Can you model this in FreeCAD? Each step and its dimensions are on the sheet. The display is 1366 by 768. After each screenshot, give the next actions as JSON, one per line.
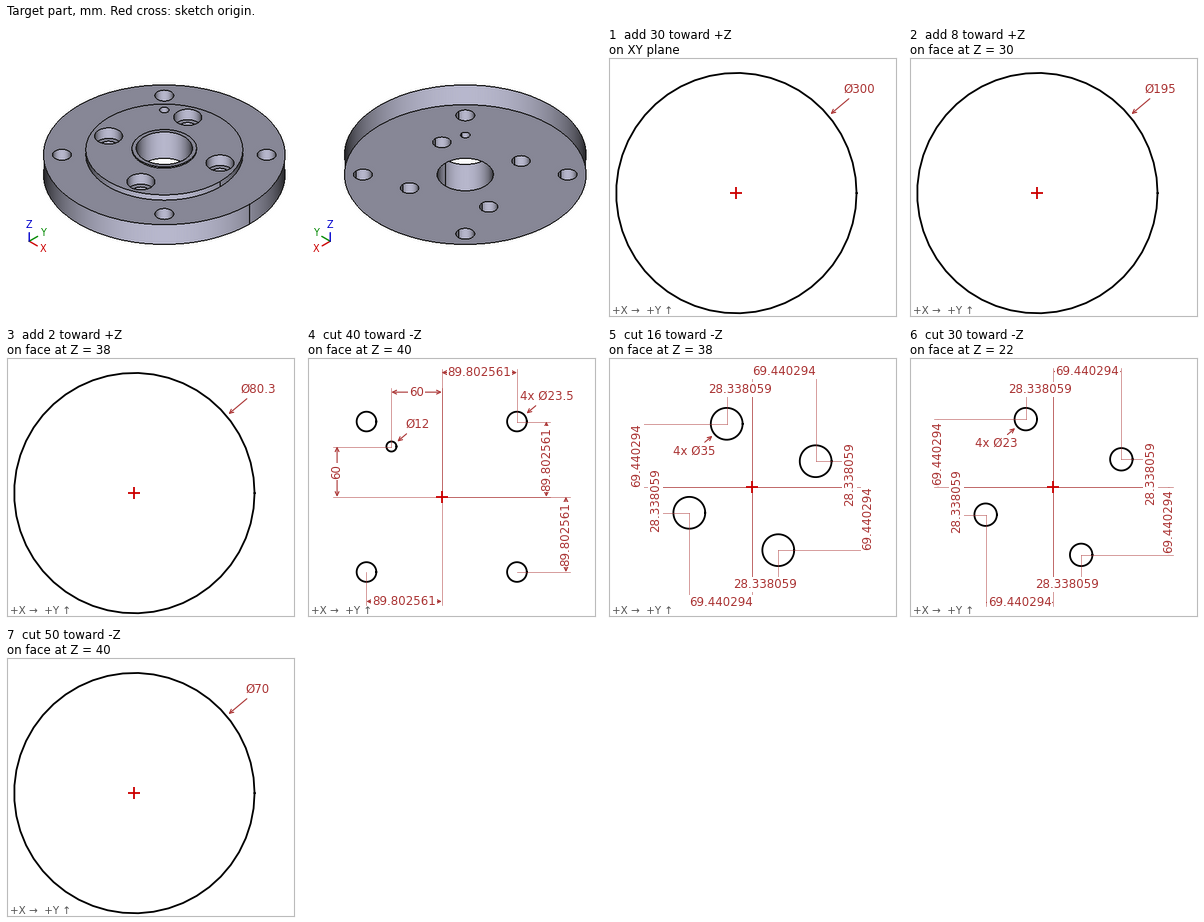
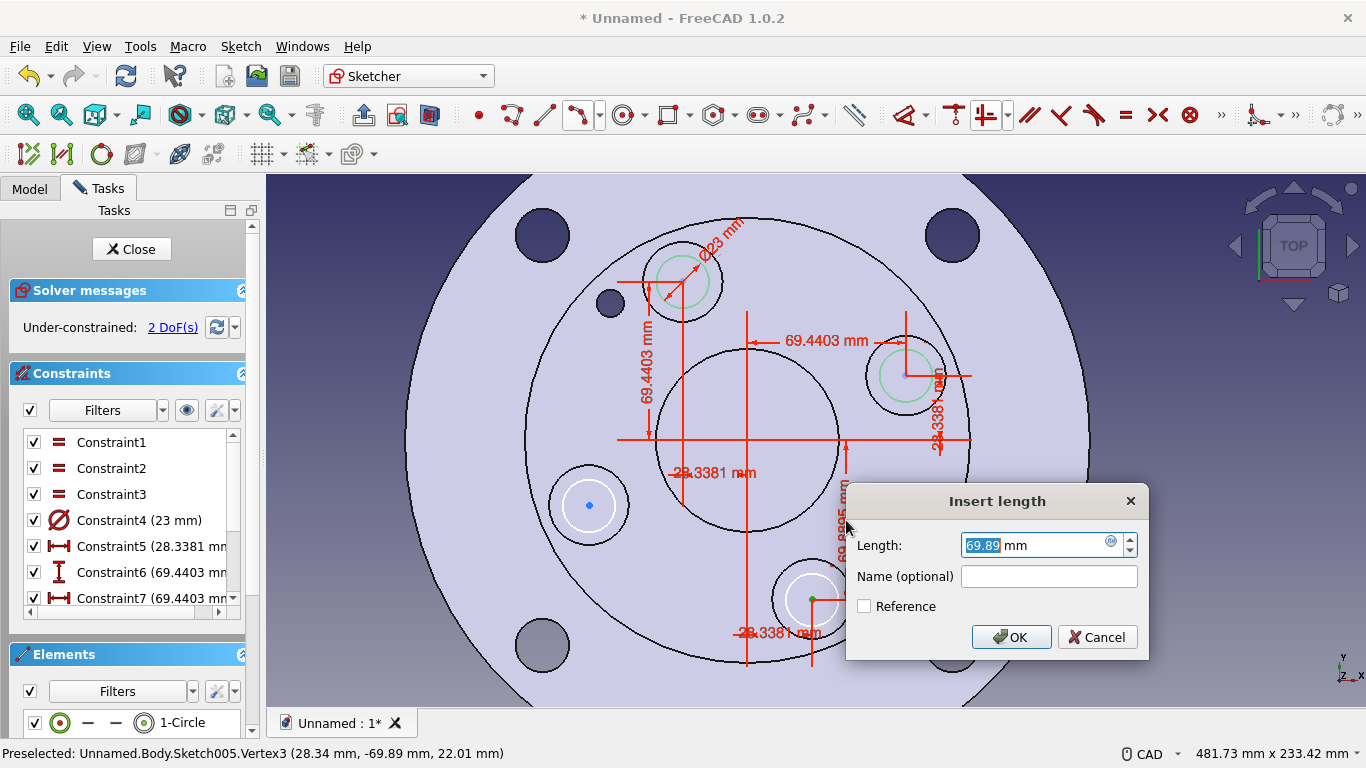
{"action": "type", "text": "69.440294"}
{"action": "key", "text": "Return"}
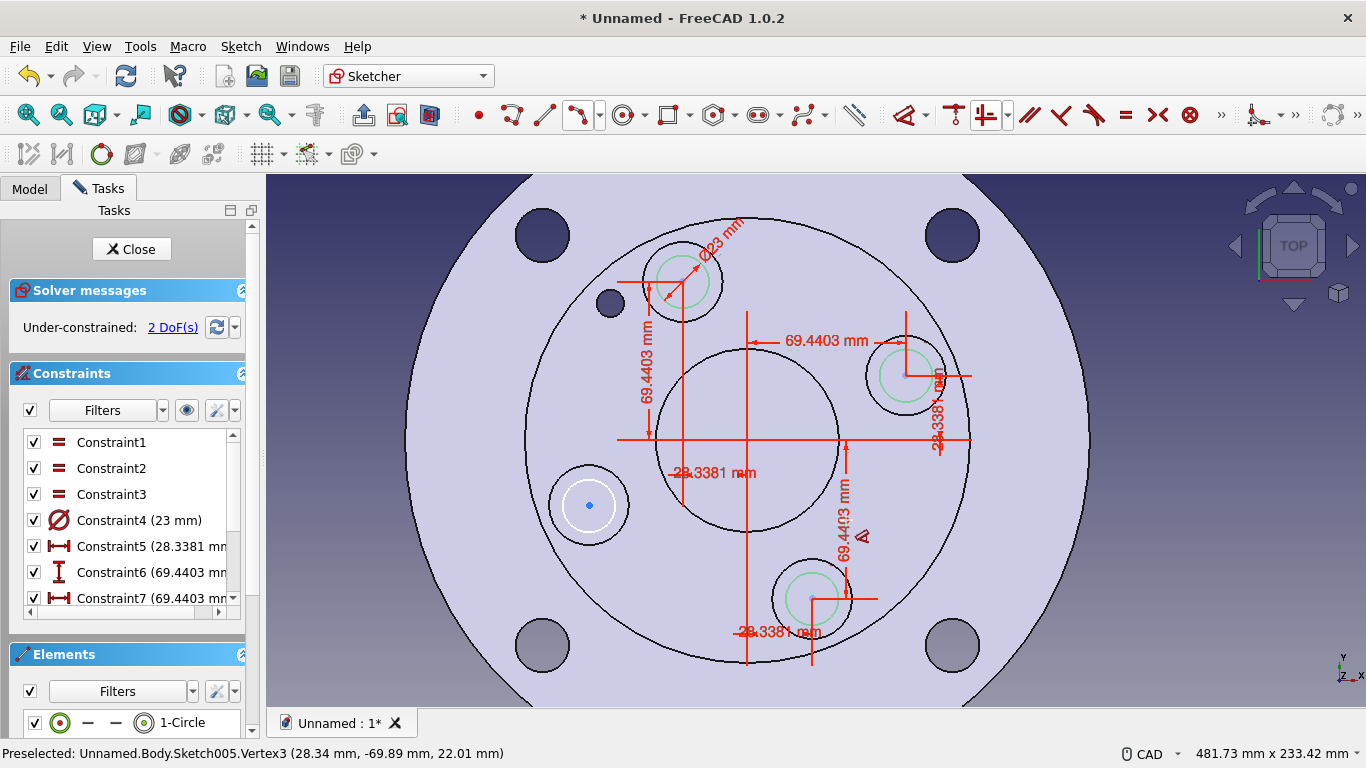
{"action": "left_click", "coordinate": [589, 506]}
{"action": "left_click", "coordinate": [668, 540]}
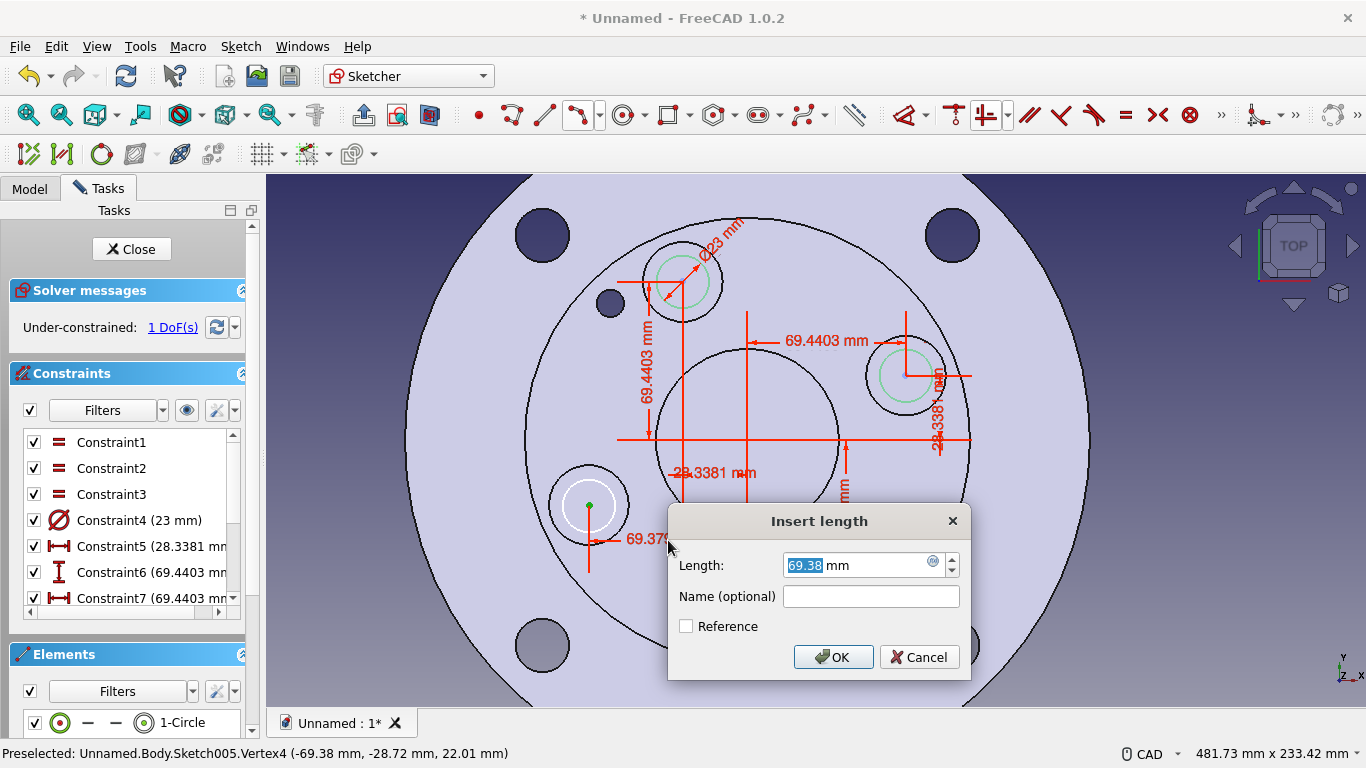
{"action": "type", "text": "69.440294"}
{"action": "key", "text": "Return"}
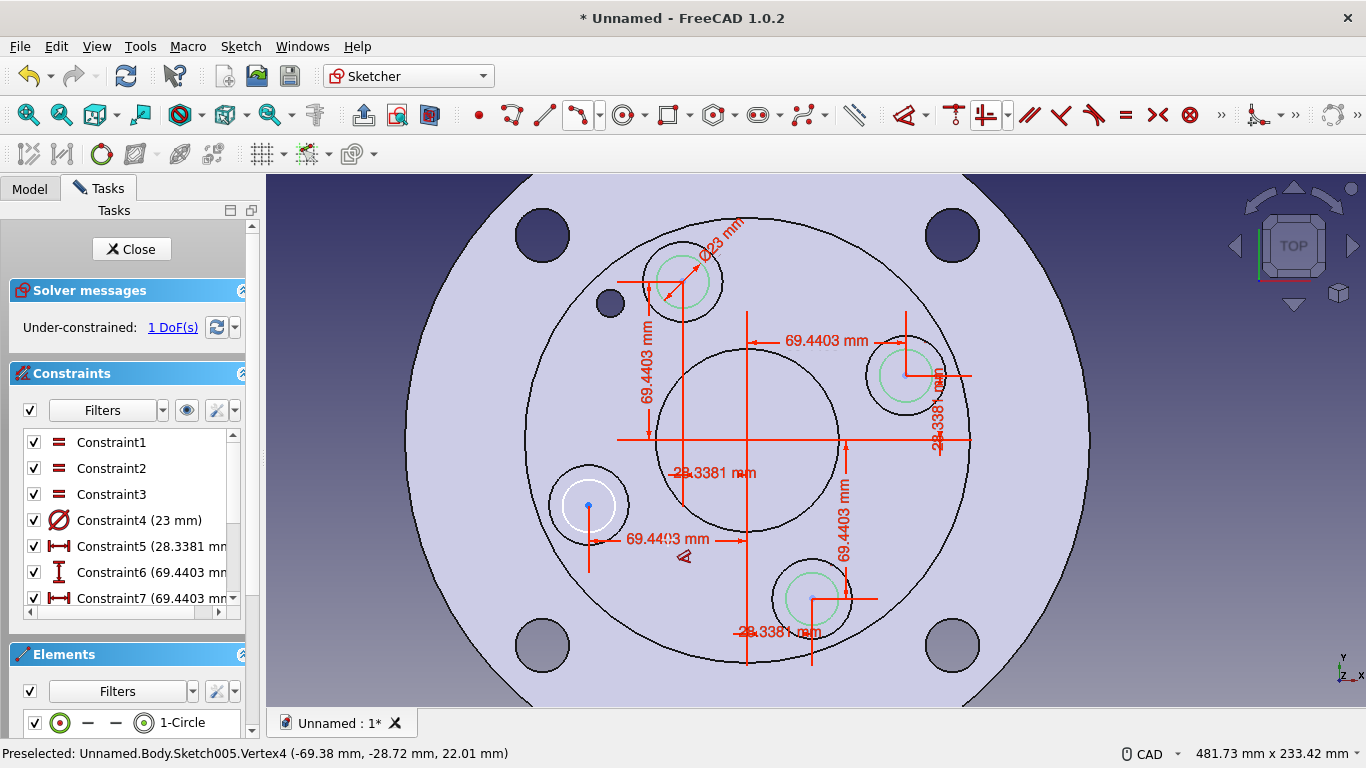
{"action": "left_click", "coordinate": [589, 506]}
{"action": "left_click", "coordinate": [555, 473]}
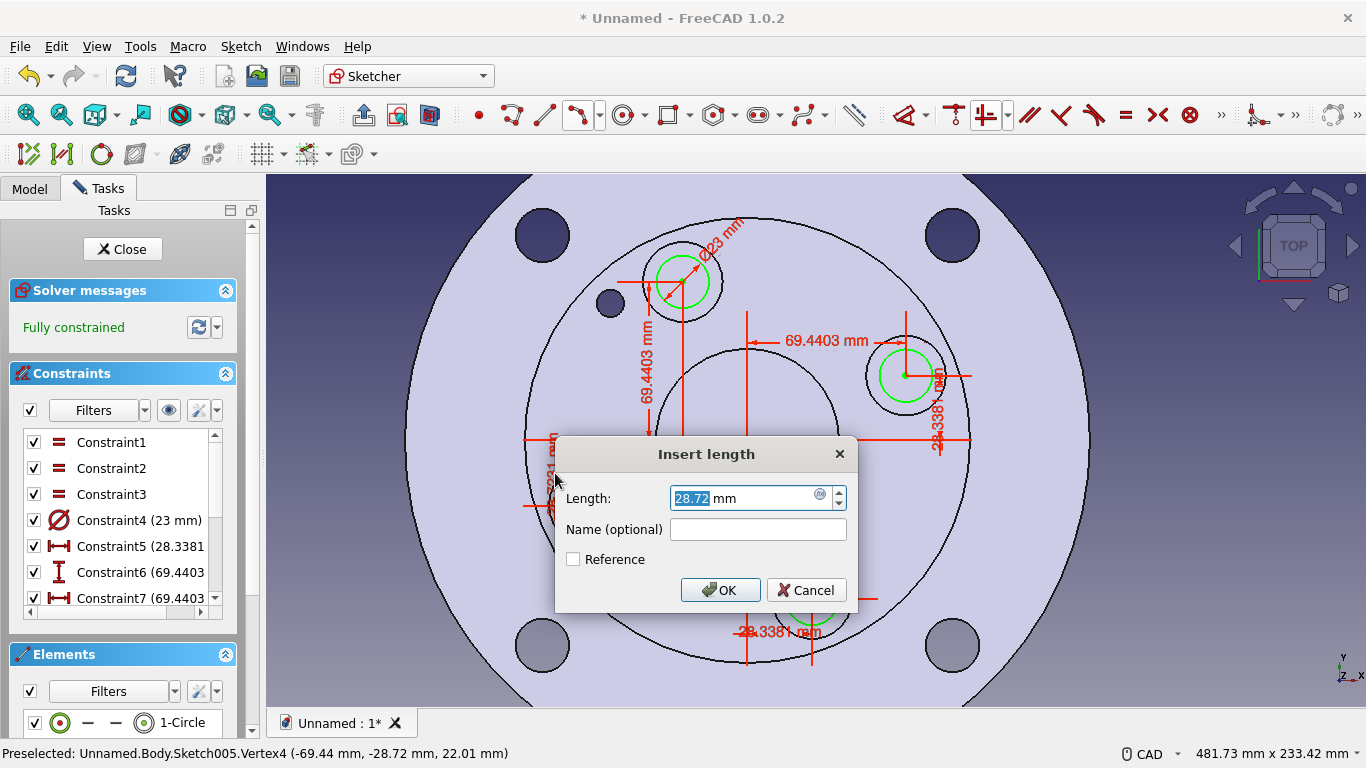
{"action": "type", "text": "28.338059"}
{"action": "key", "text": "Return"}
{"action": "key", "text": "Escape"}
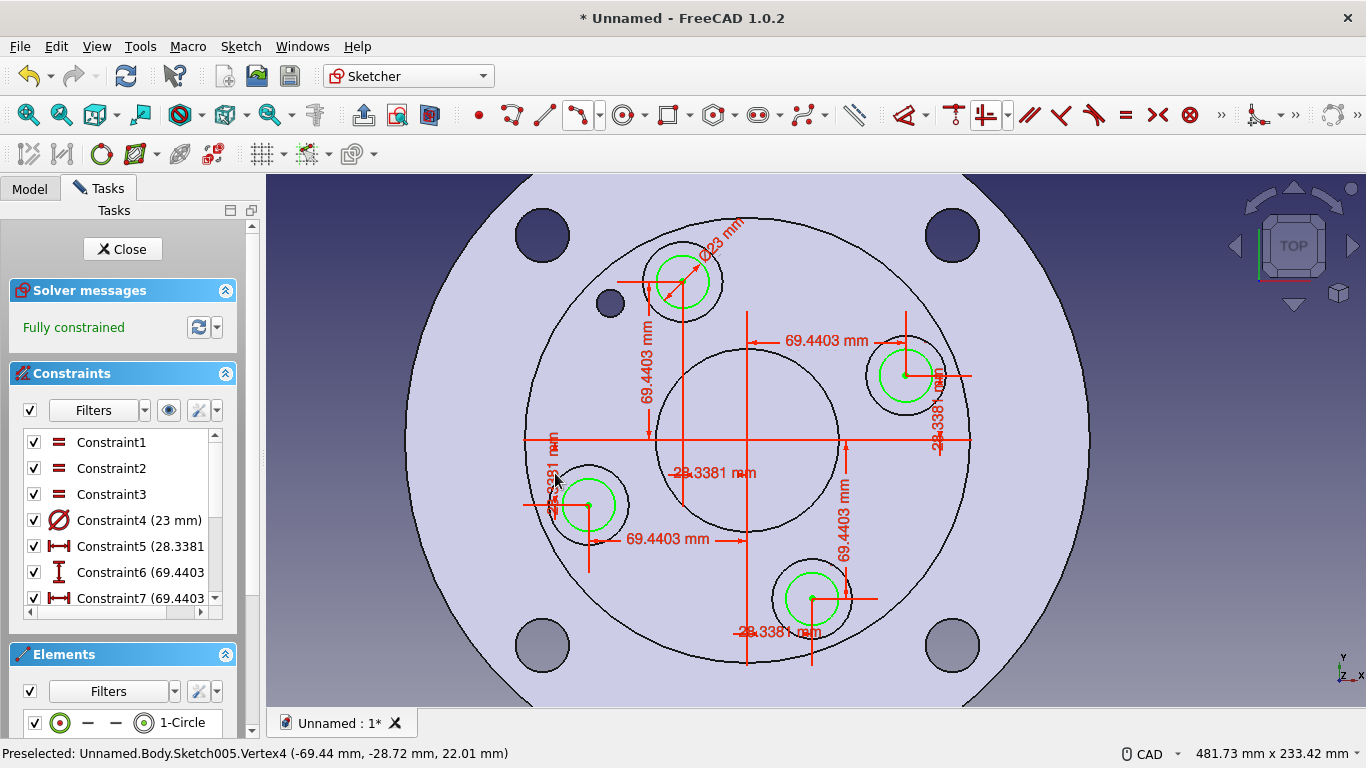
{"action": "left_click", "coordinate": [123, 249]}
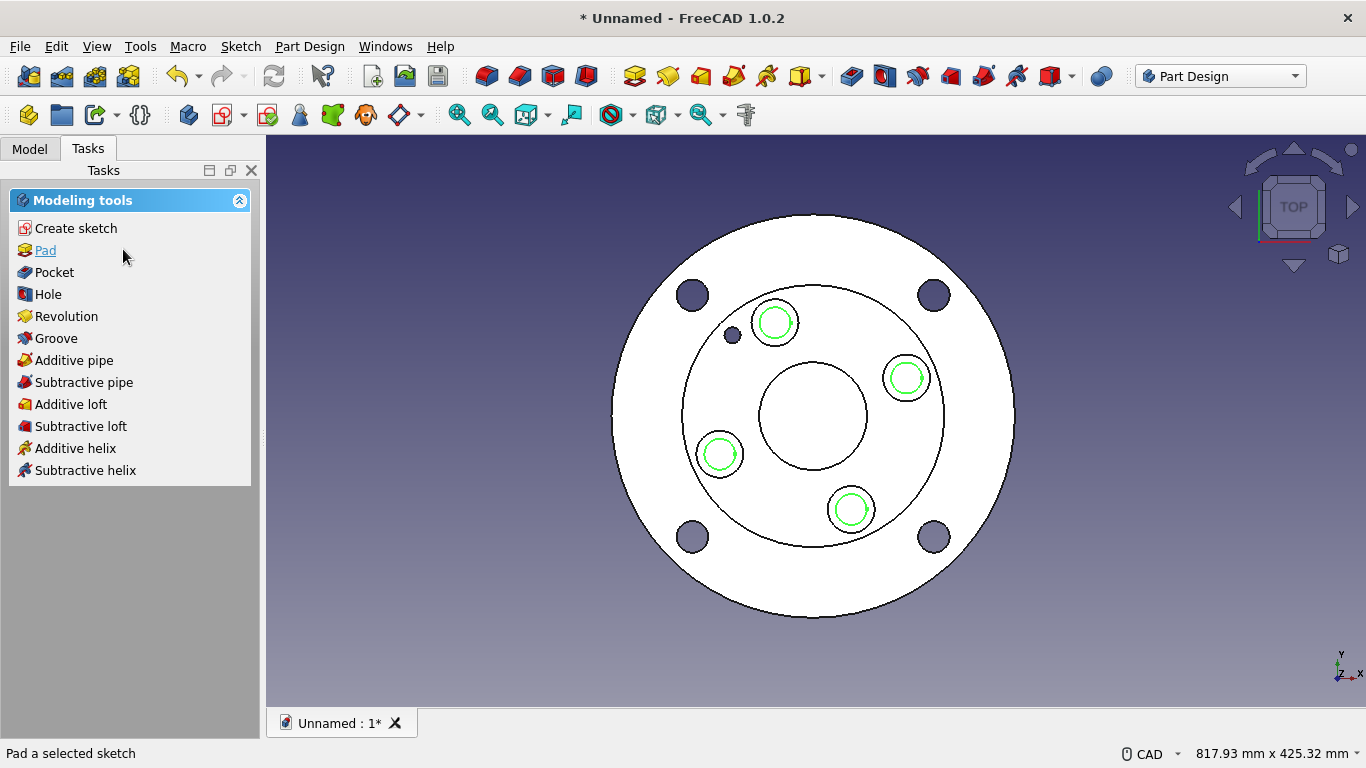
{"action": "left_click", "coordinate": [852, 76]}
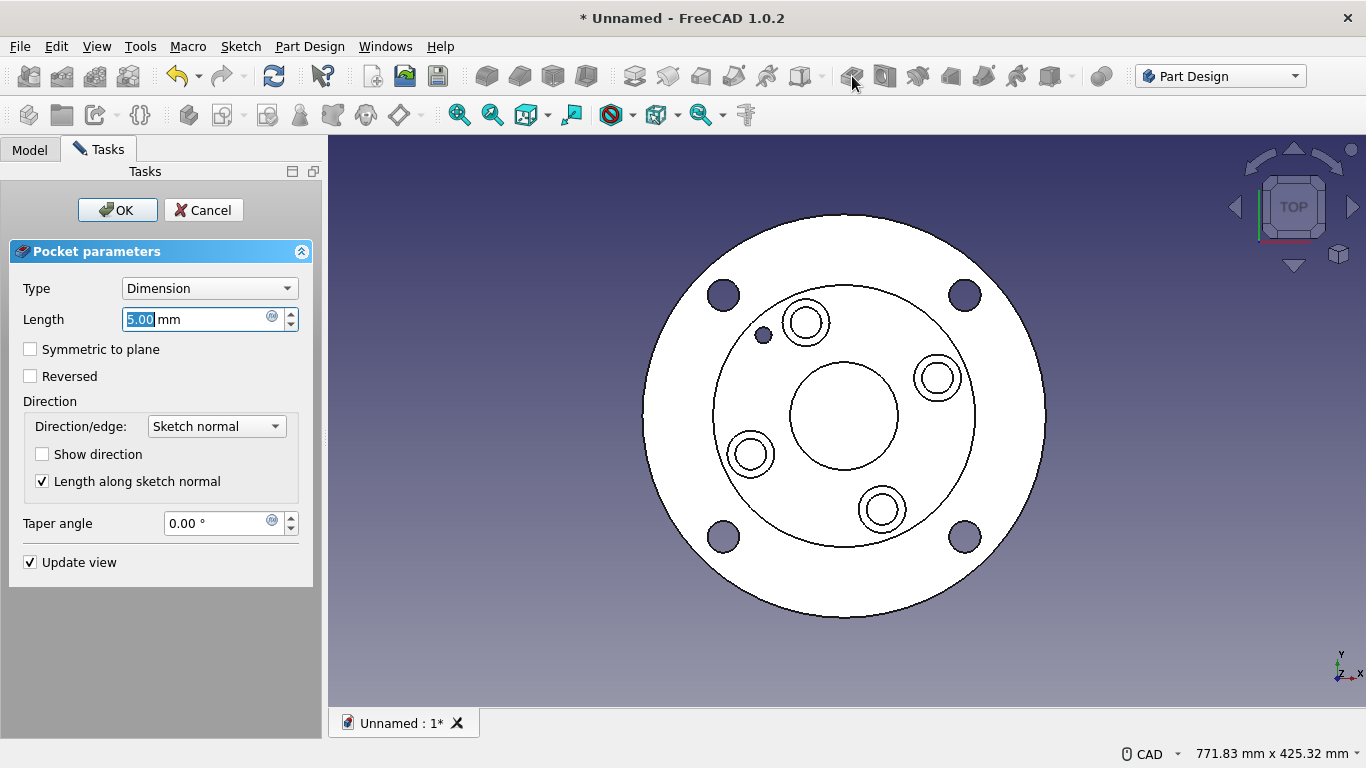
{"action": "type", "text": "30"}
{"action": "key", "text": "Tab"}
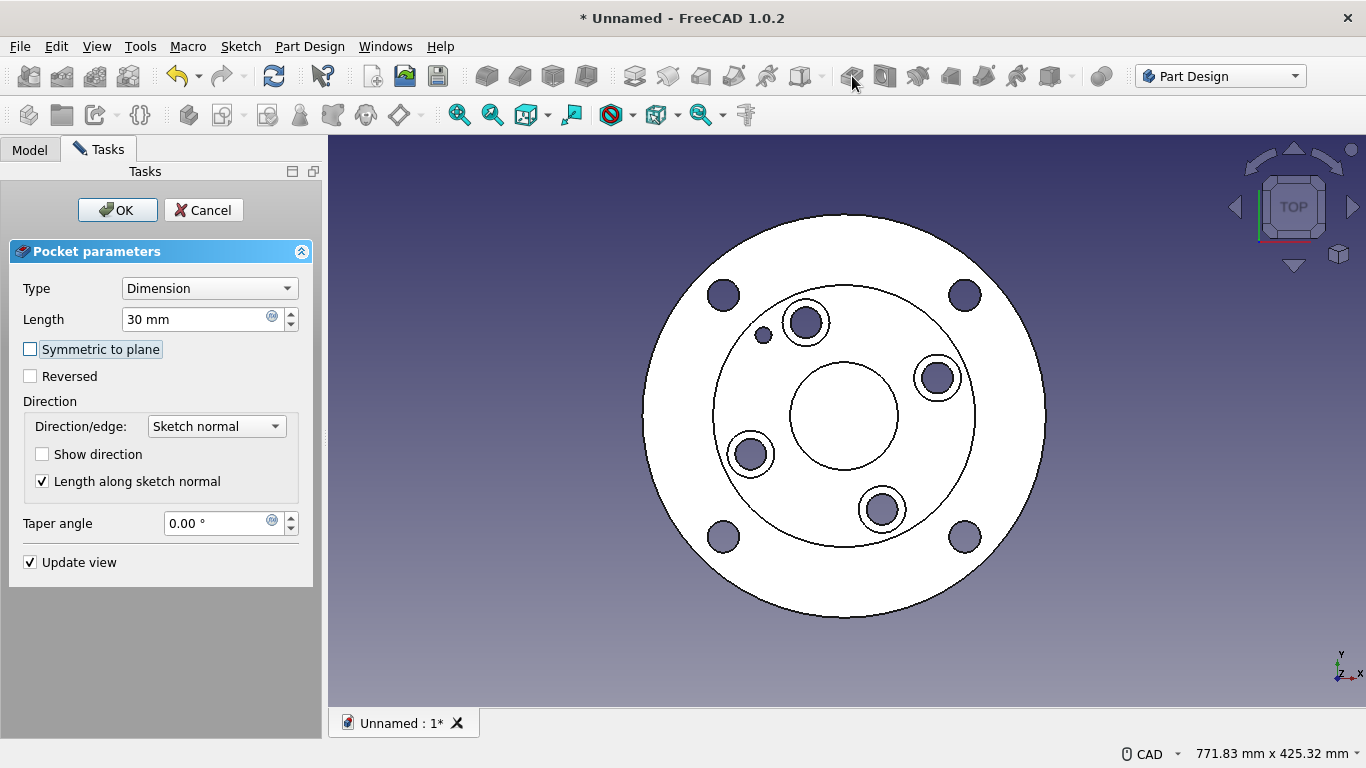
{"action": "left_click", "coordinate": [118, 210]}